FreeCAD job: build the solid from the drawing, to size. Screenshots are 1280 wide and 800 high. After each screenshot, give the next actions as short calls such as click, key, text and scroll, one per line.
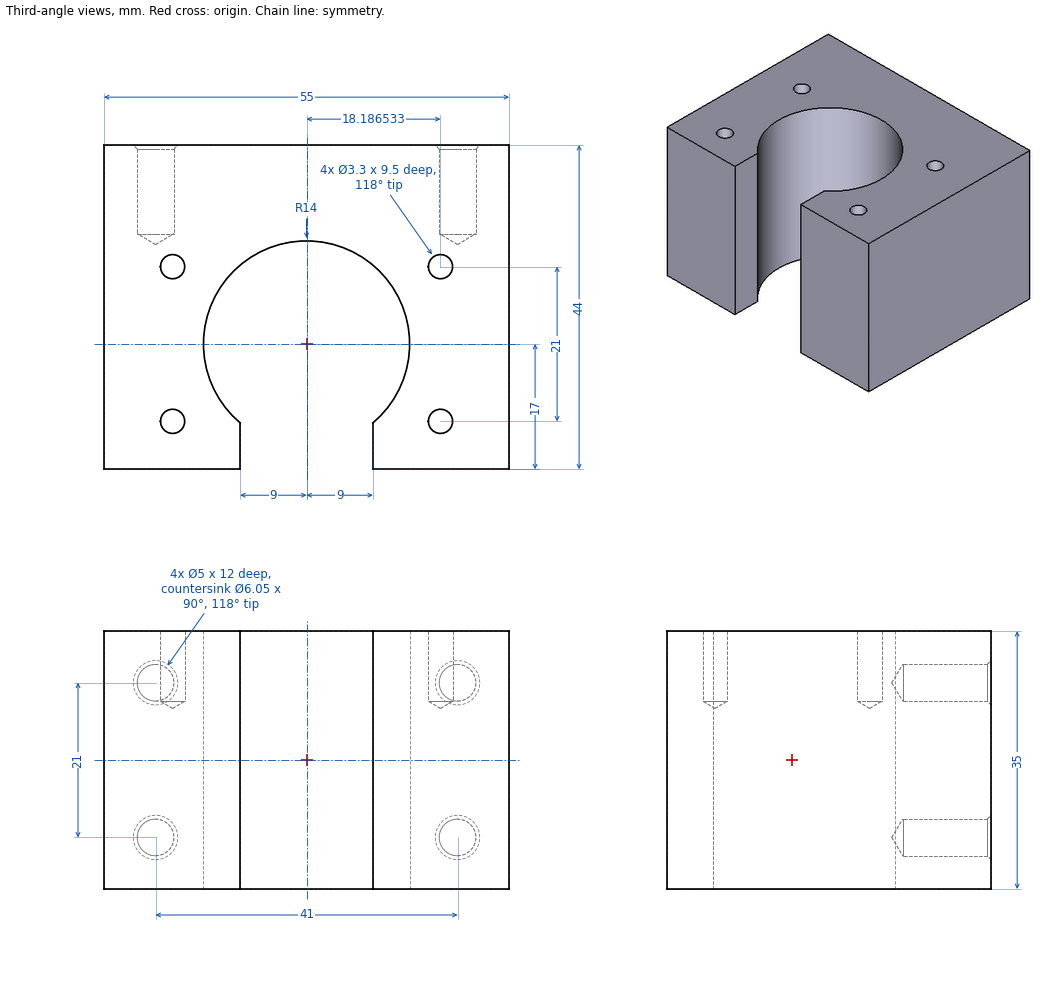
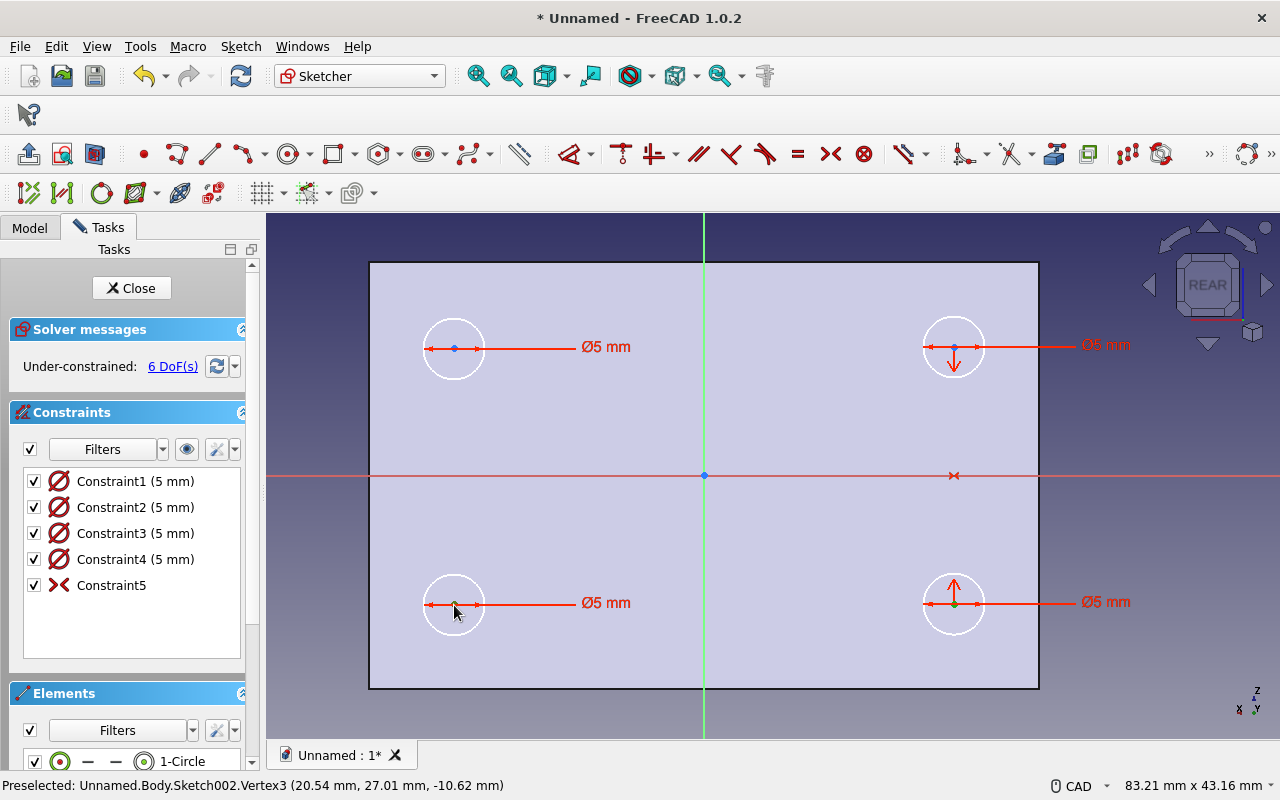
click(704, 677)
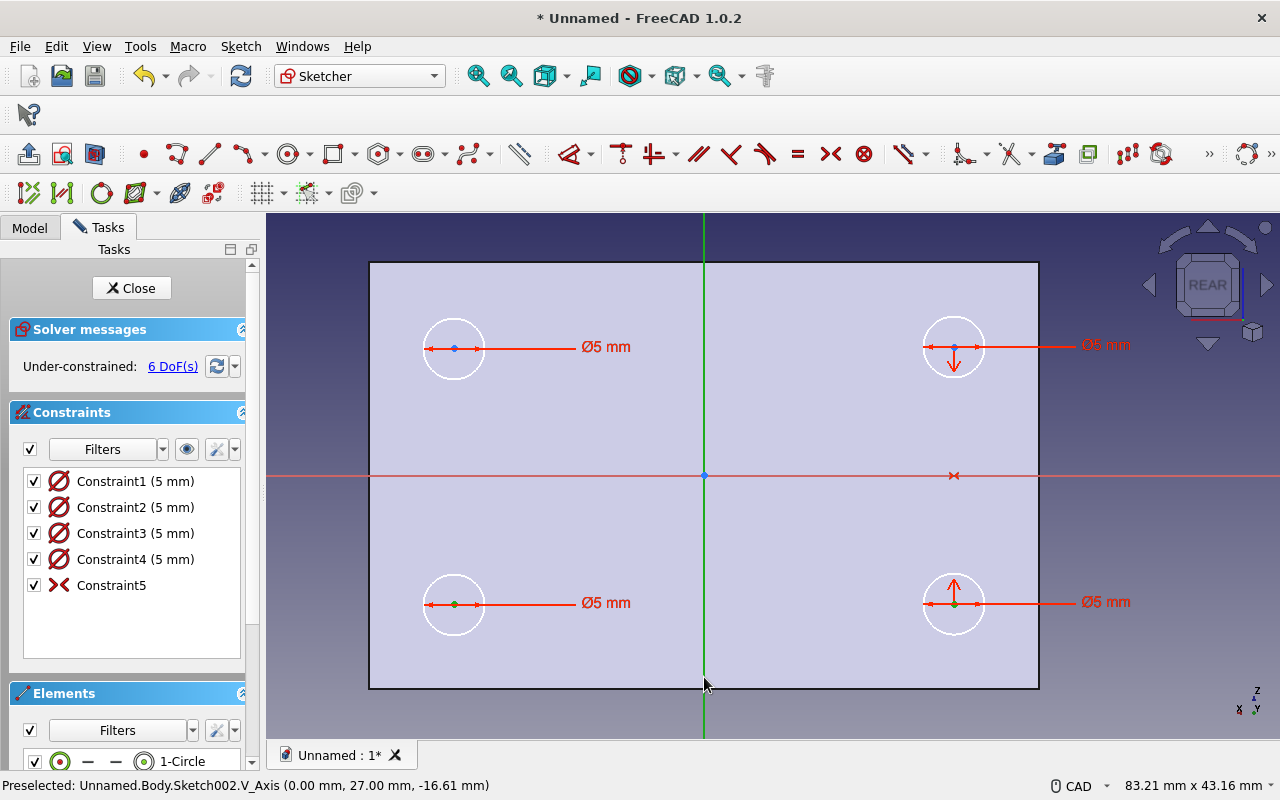
click(831, 154)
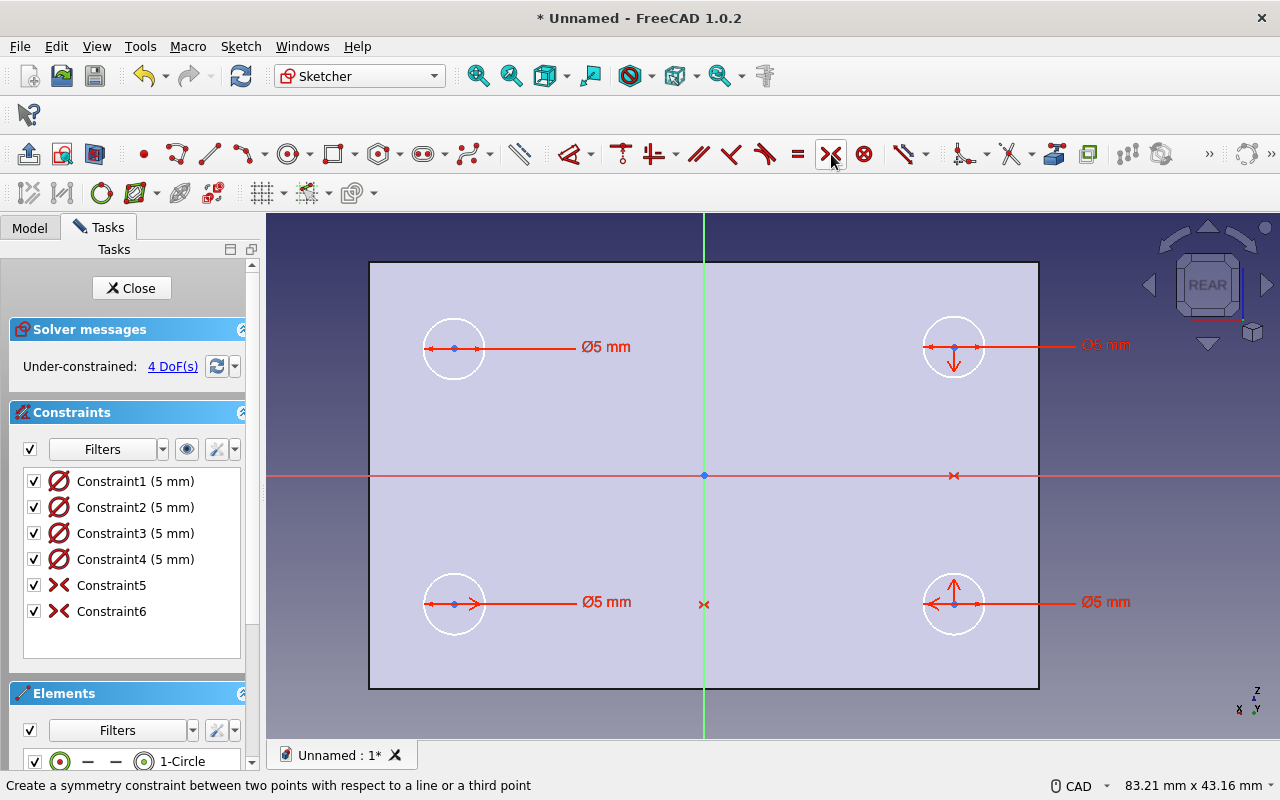
click(954, 347)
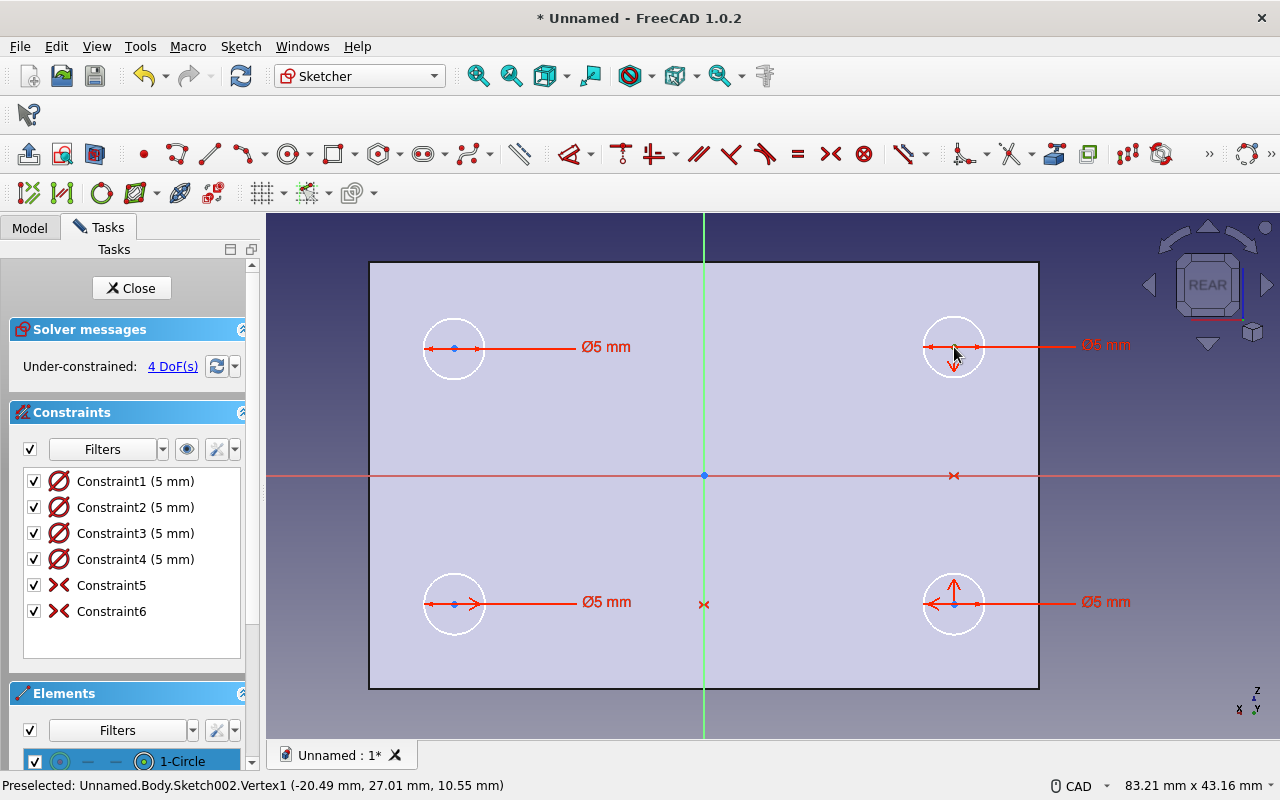
click(454, 349)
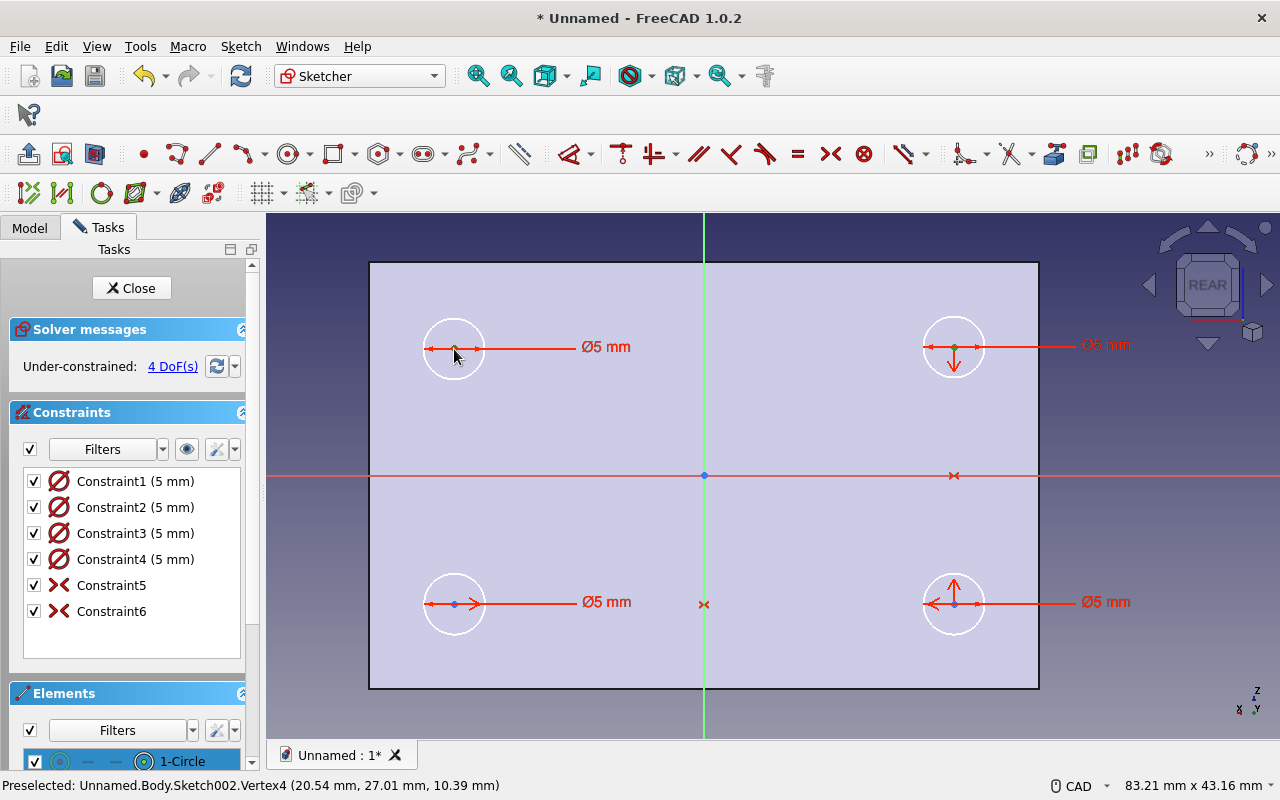
click(704, 677)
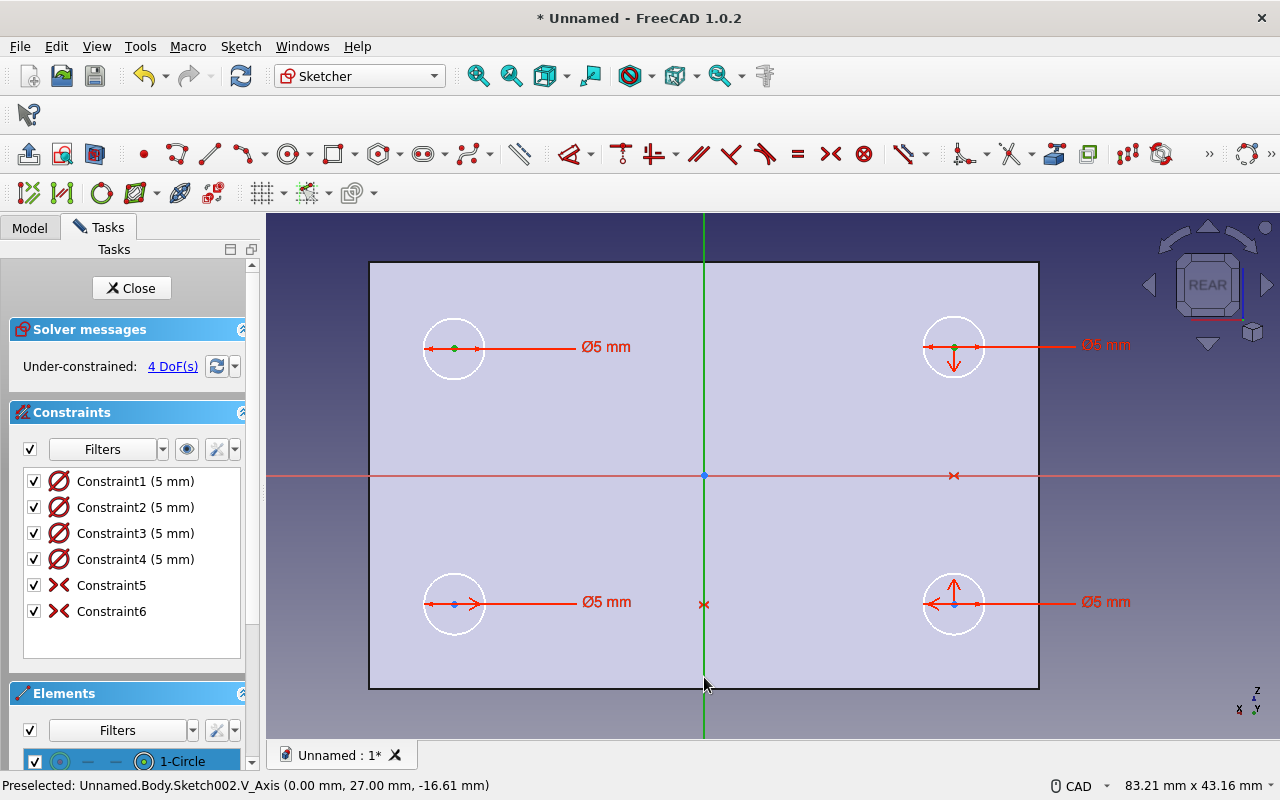
click(831, 154)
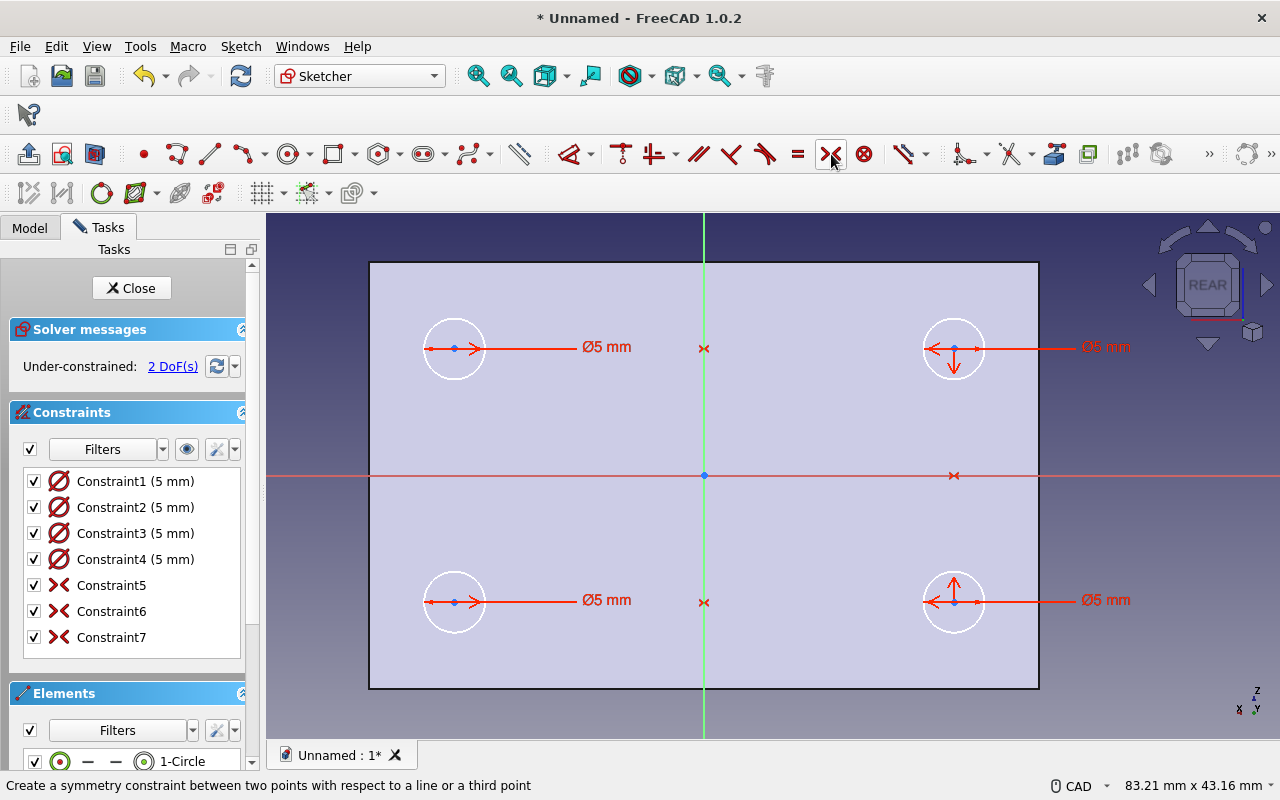
click(568, 154)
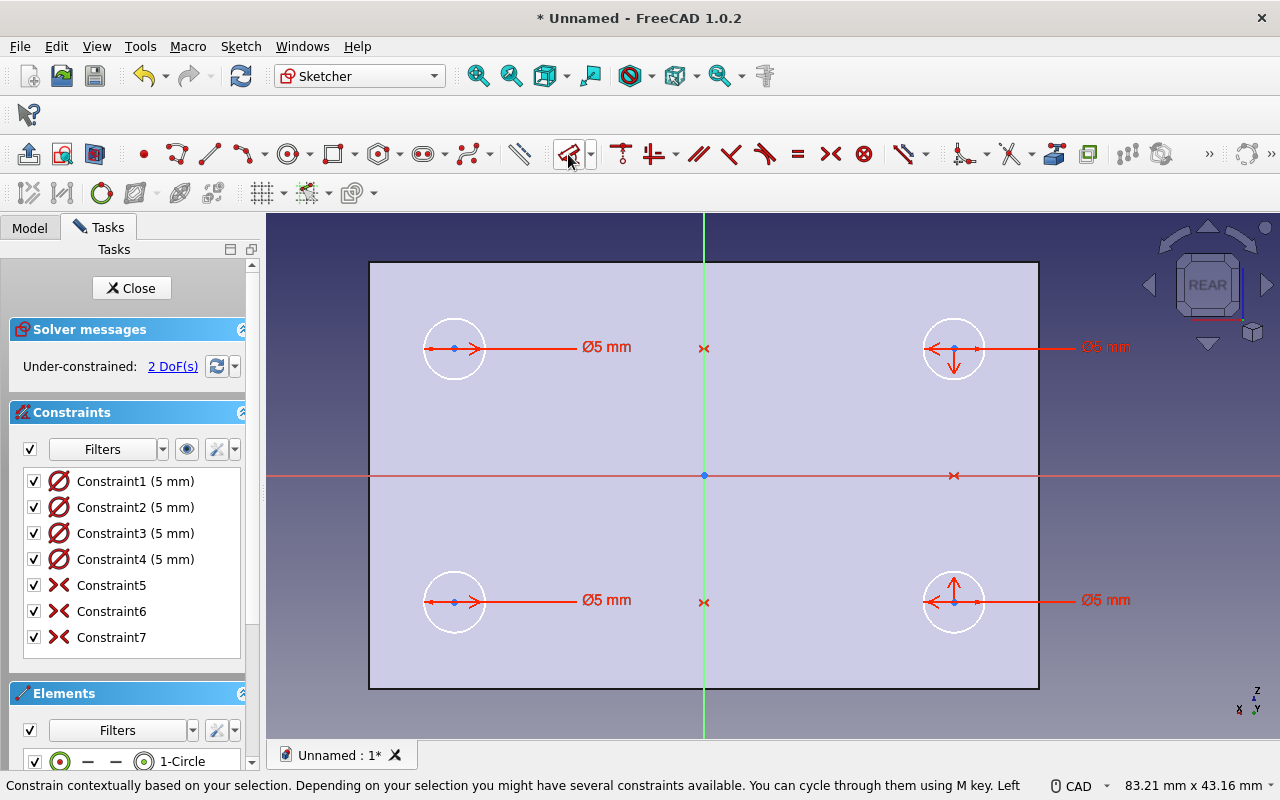
click(954, 349)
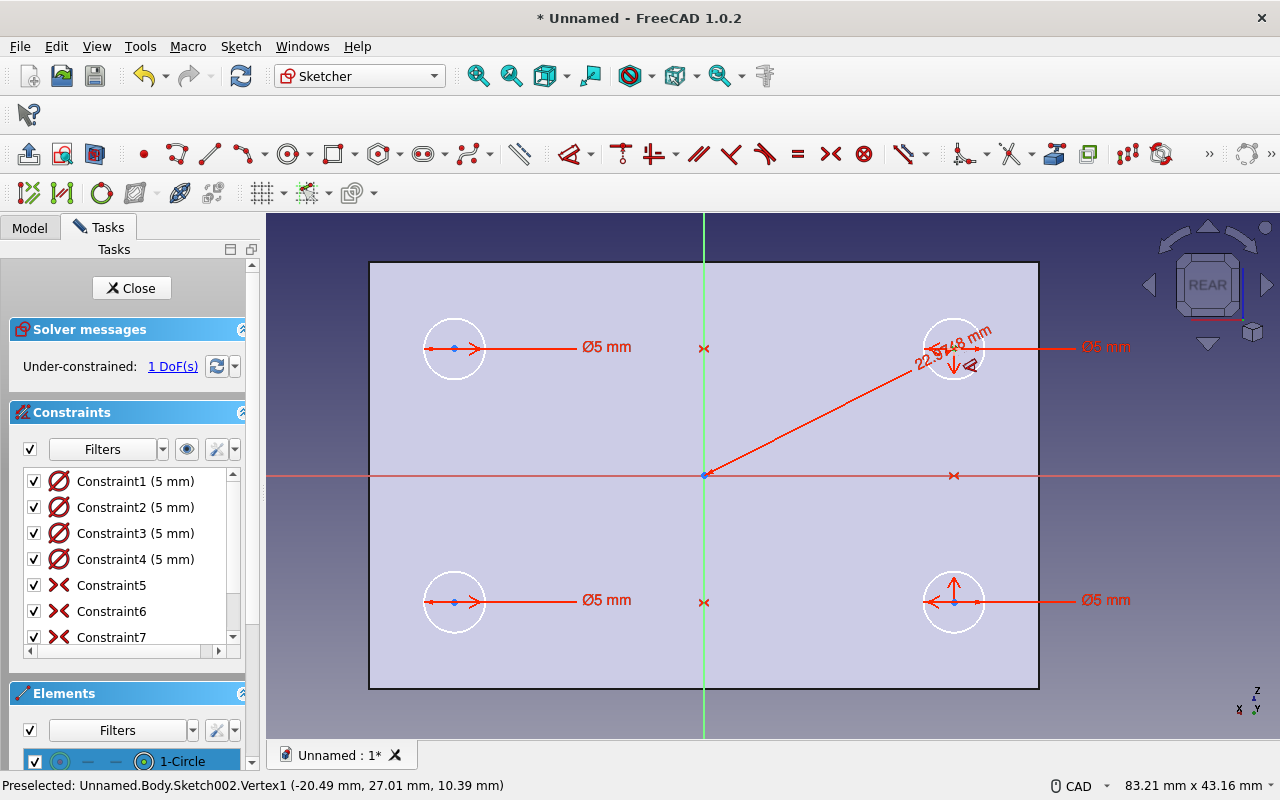
click(954, 602)
click(988, 417)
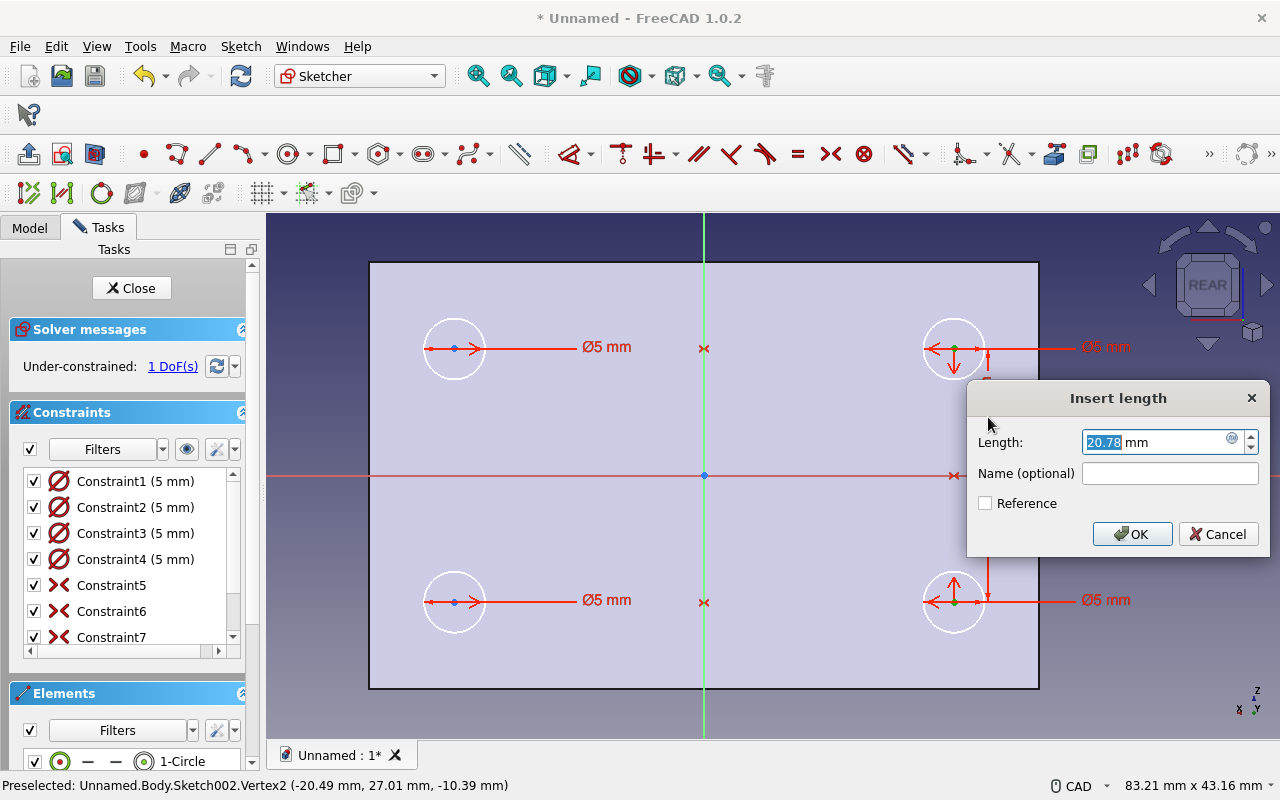
text(21)
key(Return)